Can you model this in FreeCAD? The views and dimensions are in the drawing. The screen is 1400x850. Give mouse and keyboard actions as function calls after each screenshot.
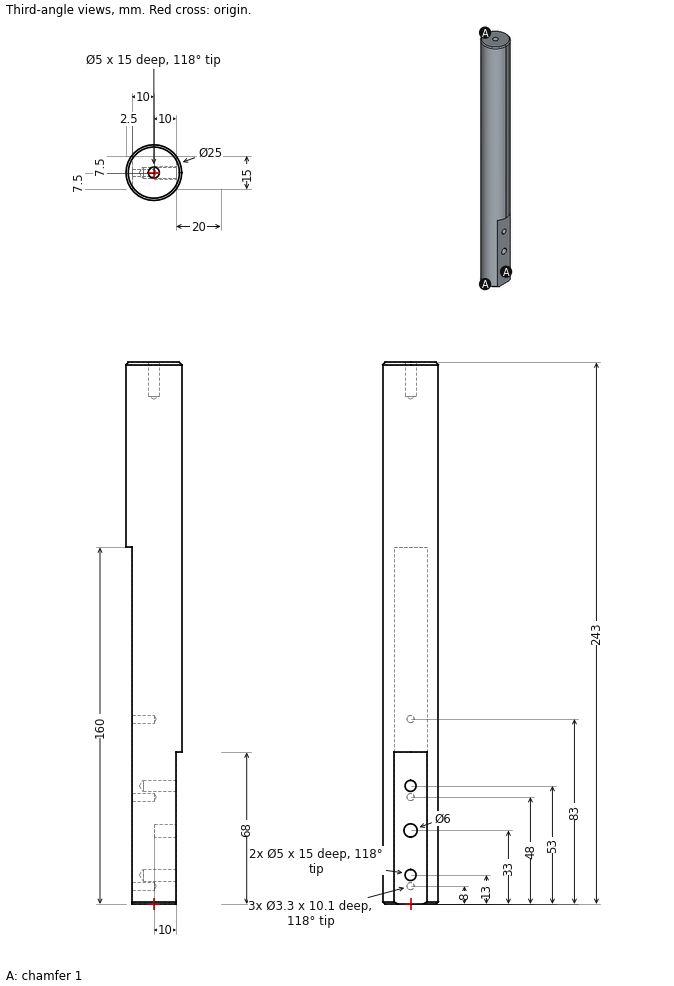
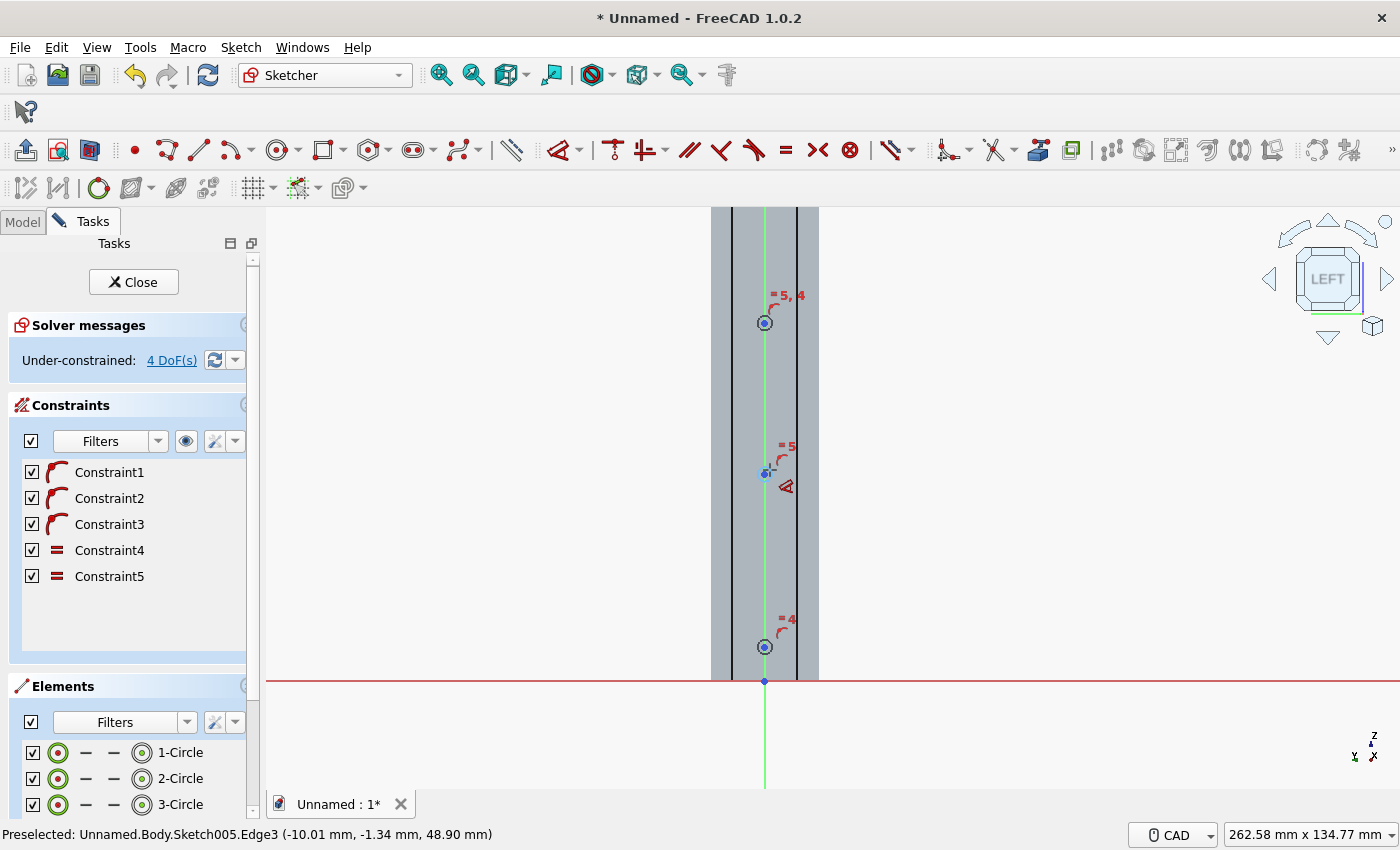
scroll(770, 642, up, 6)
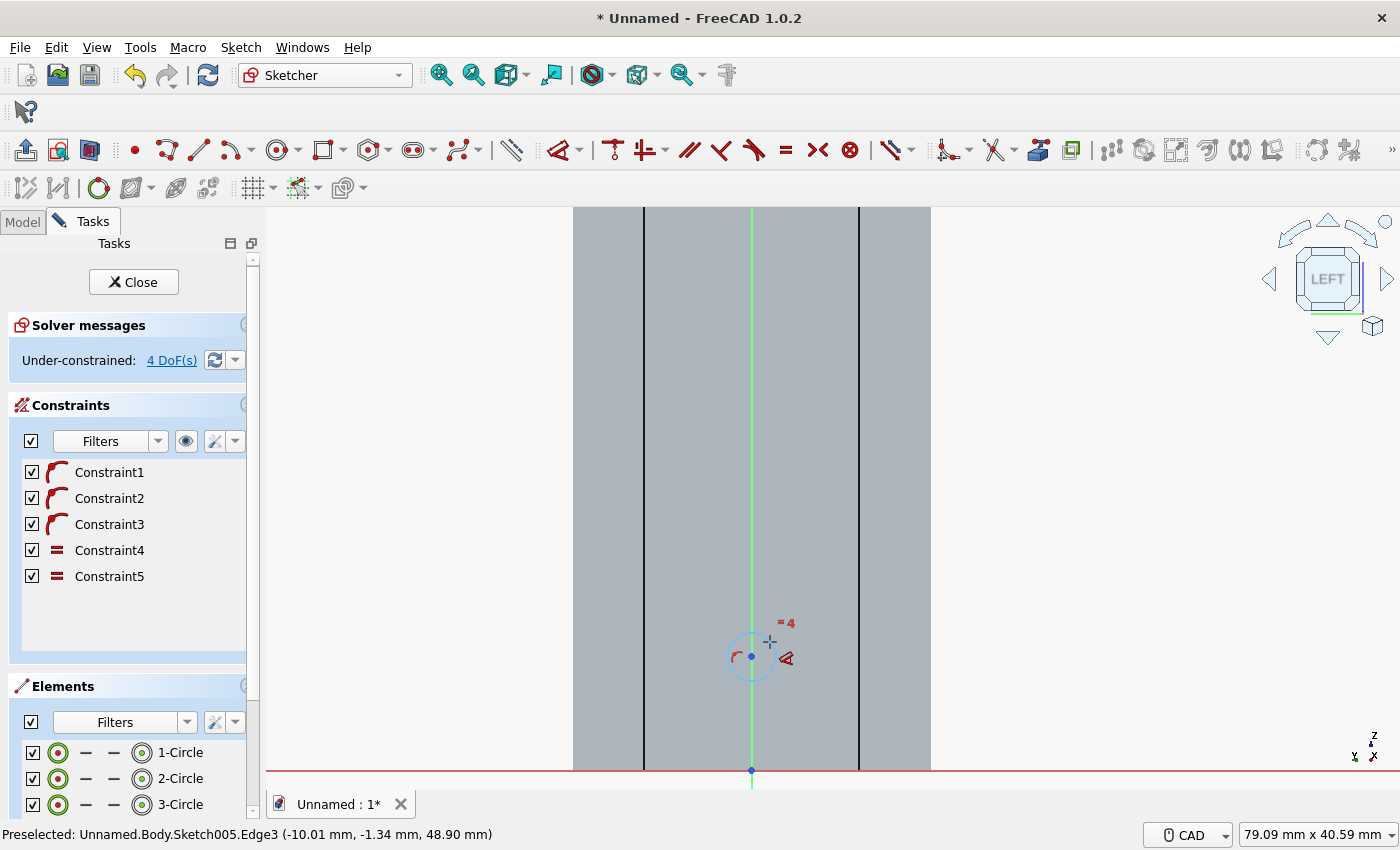
click(769, 640)
click(792, 617)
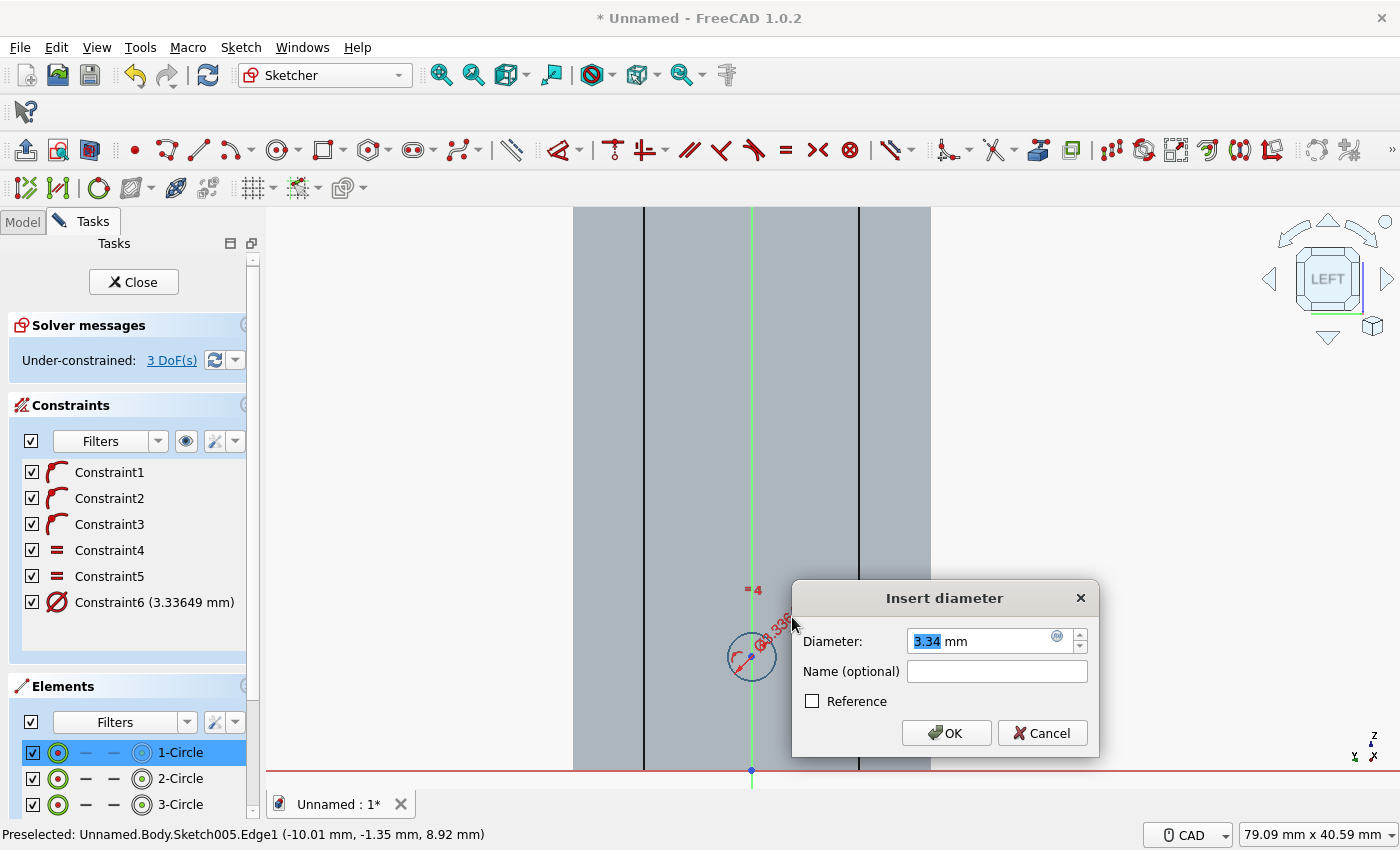
text(3.3)
key(Return)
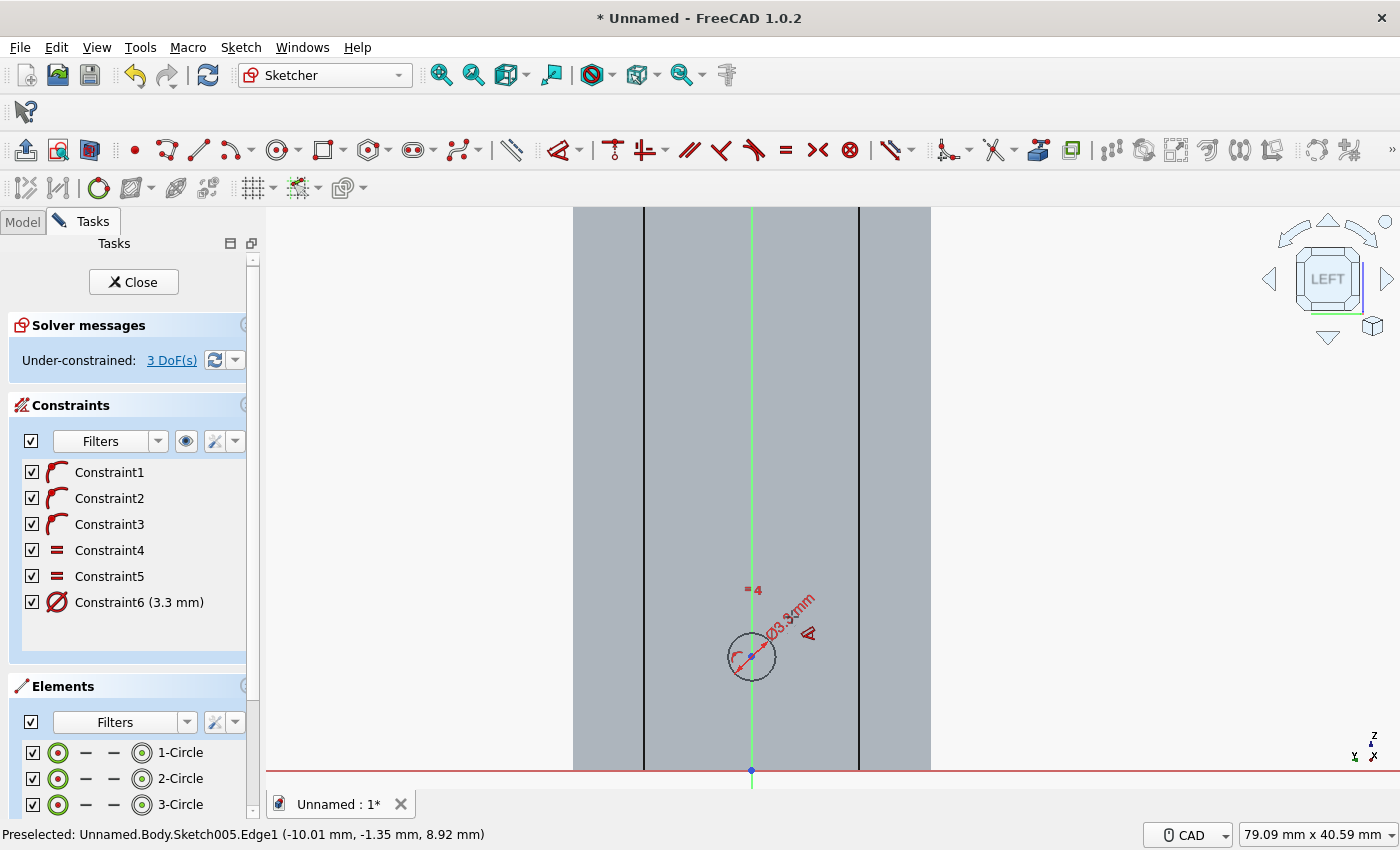
click(752, 657)
click(786, 709)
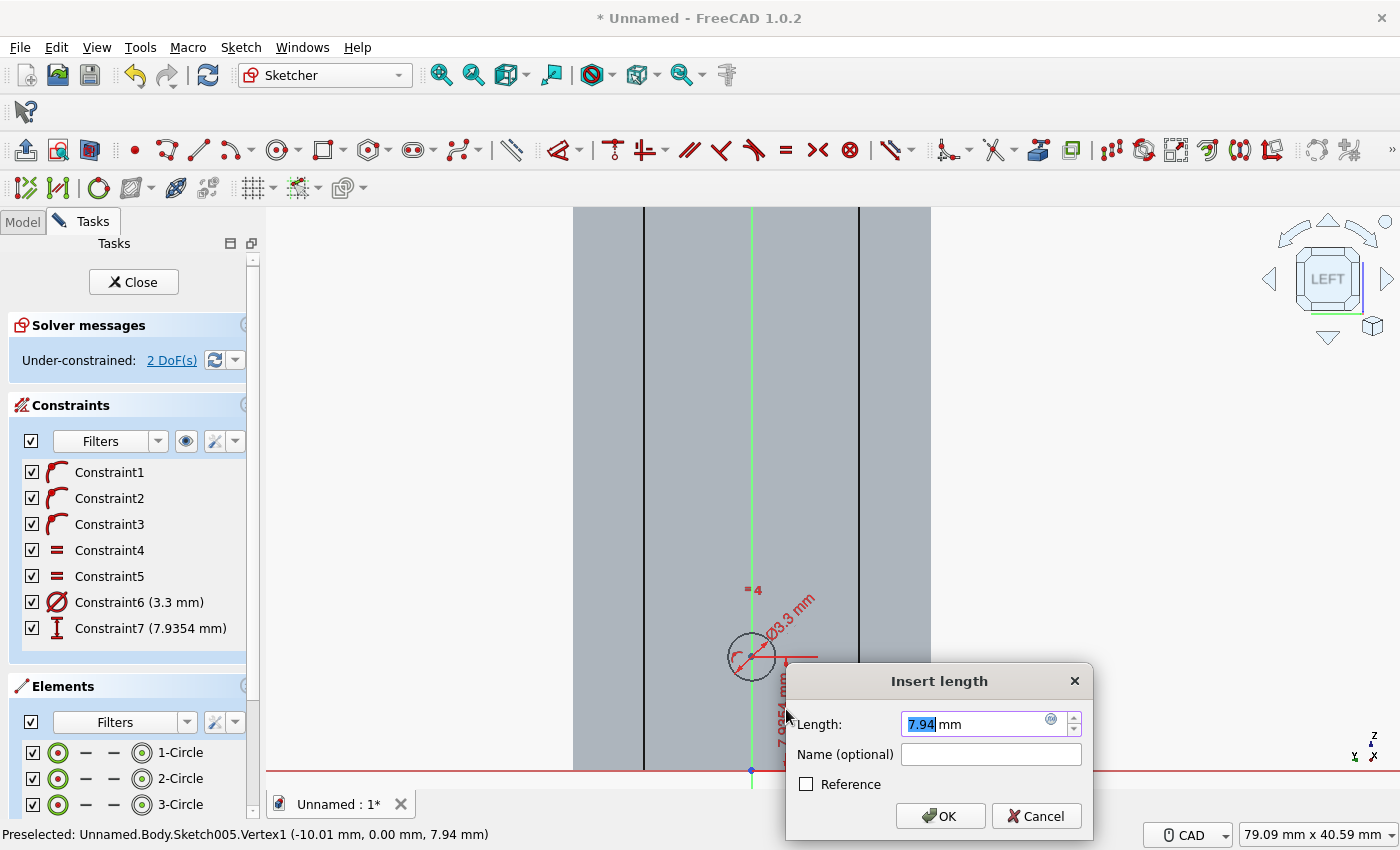
text(8)
key(Return)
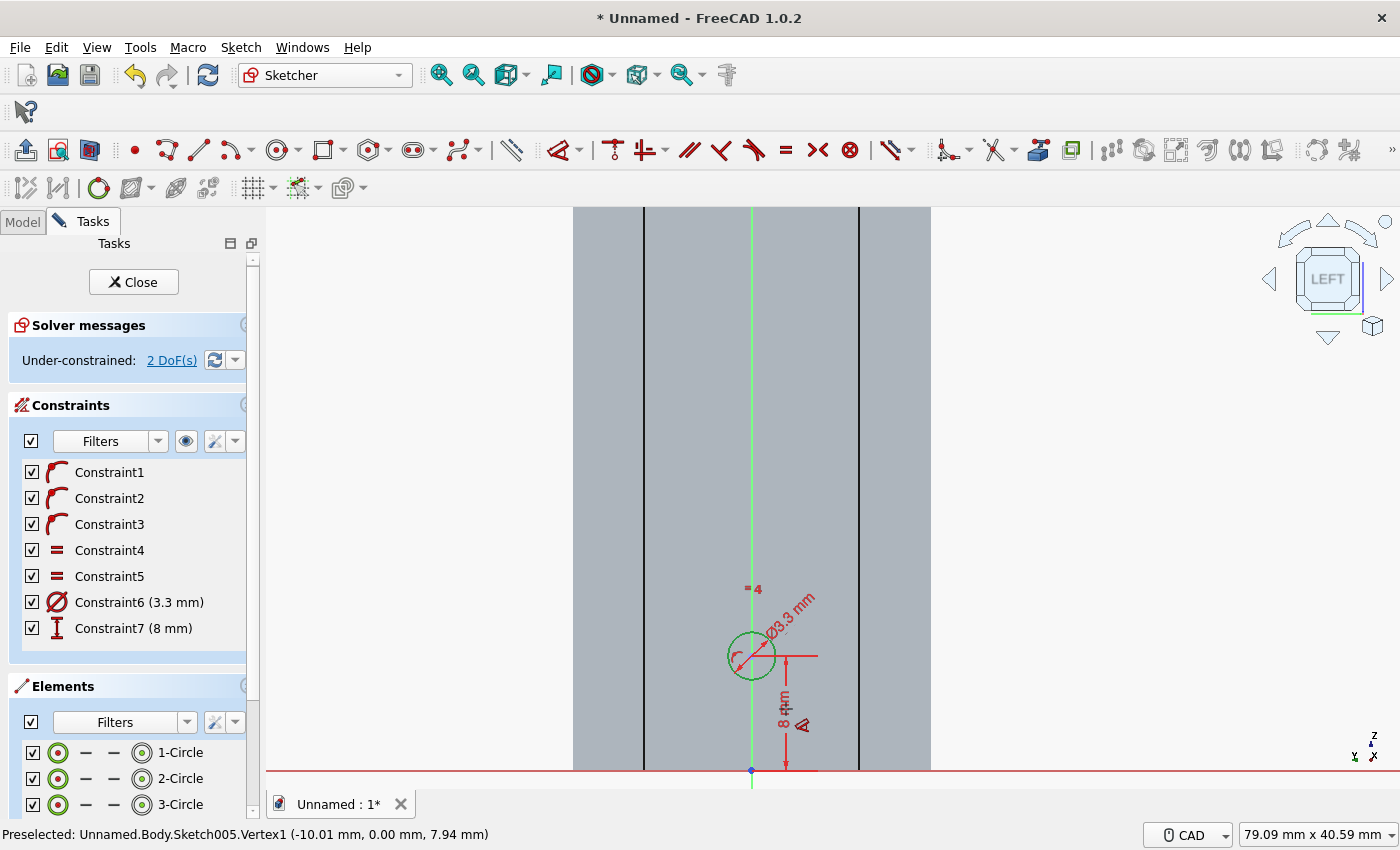
scroll(770, 642, down, 6)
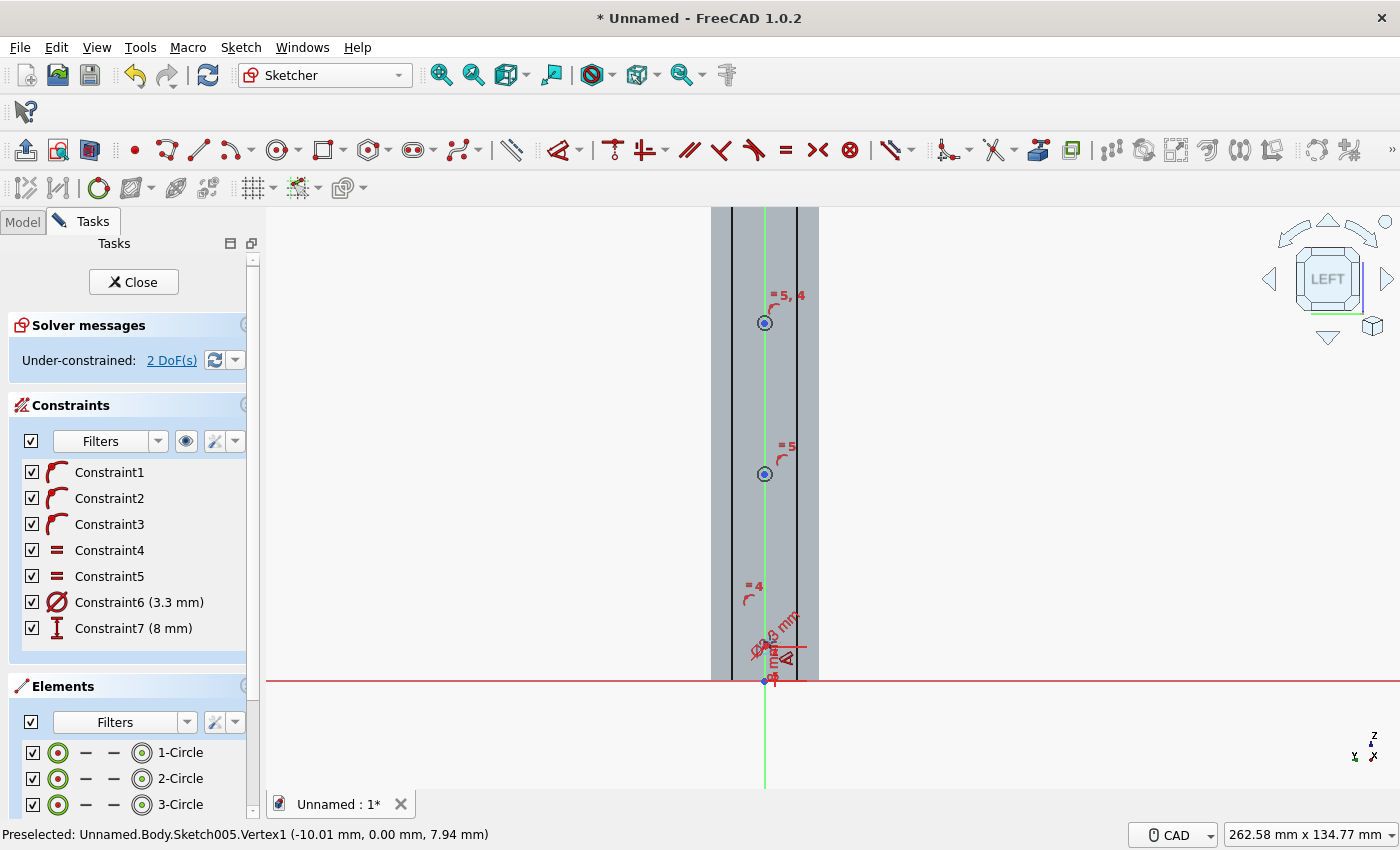
click(765, 323)
click(799, 502)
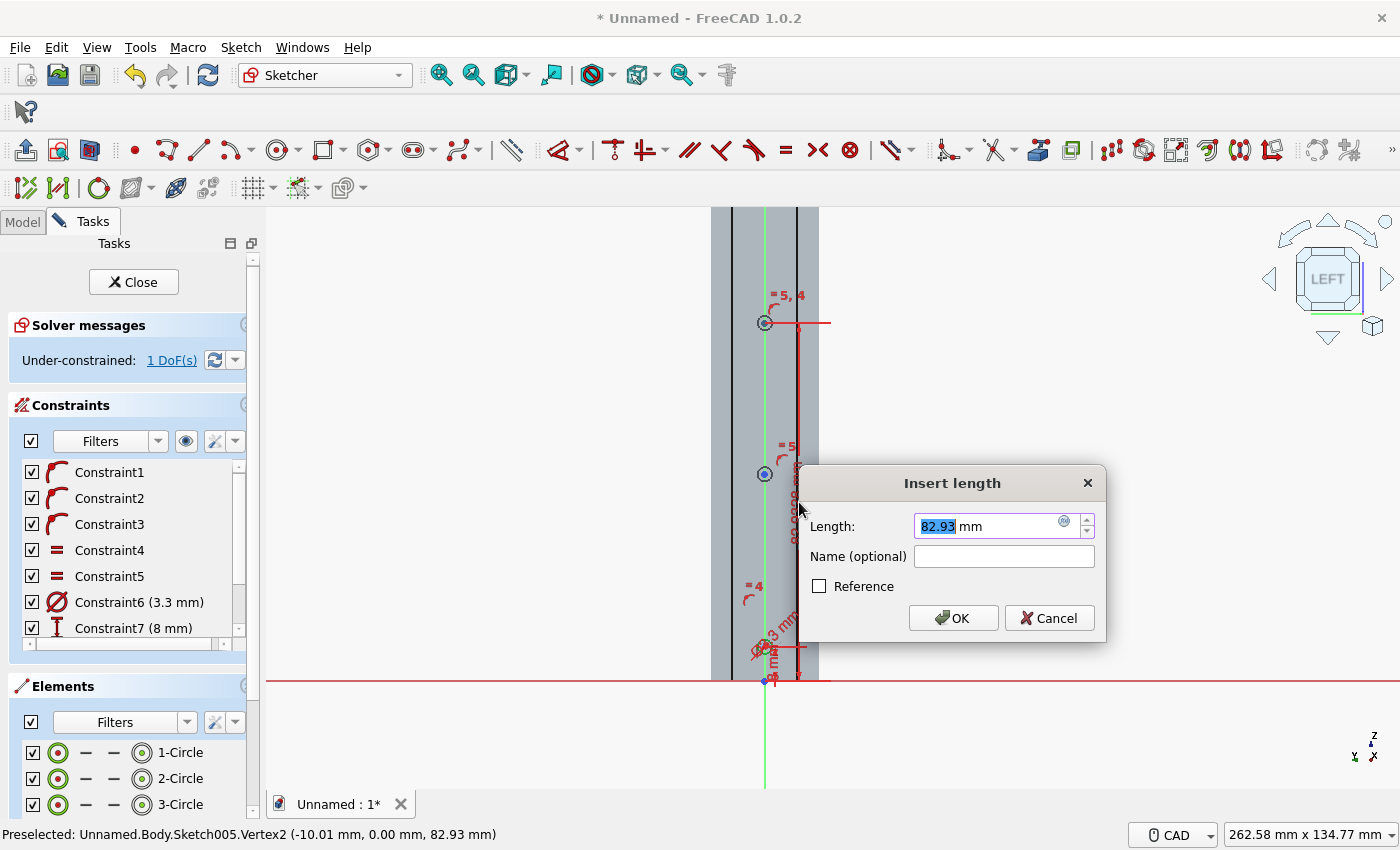
text(83)
key(Return)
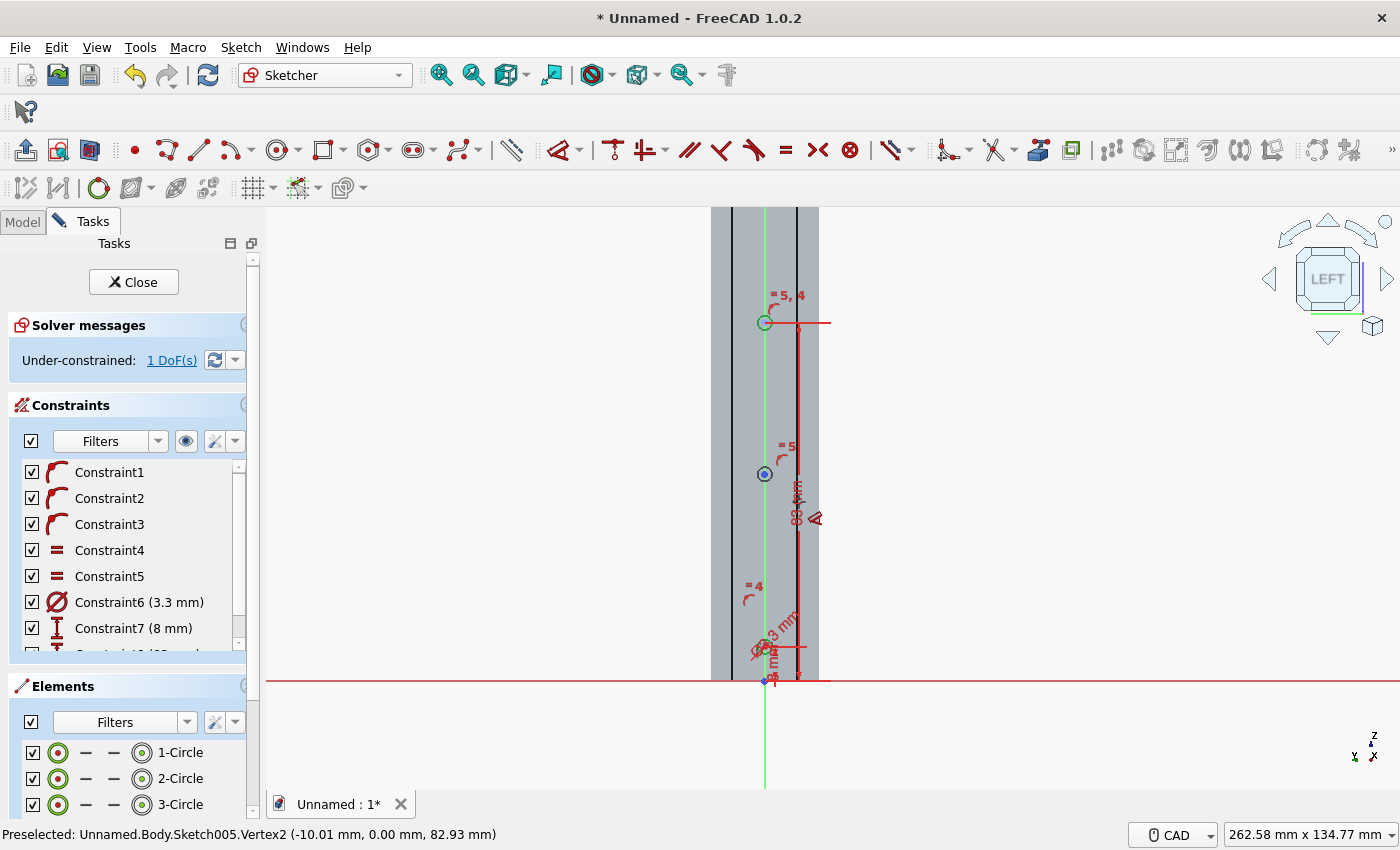
click(765, 474)
click(799, 578)